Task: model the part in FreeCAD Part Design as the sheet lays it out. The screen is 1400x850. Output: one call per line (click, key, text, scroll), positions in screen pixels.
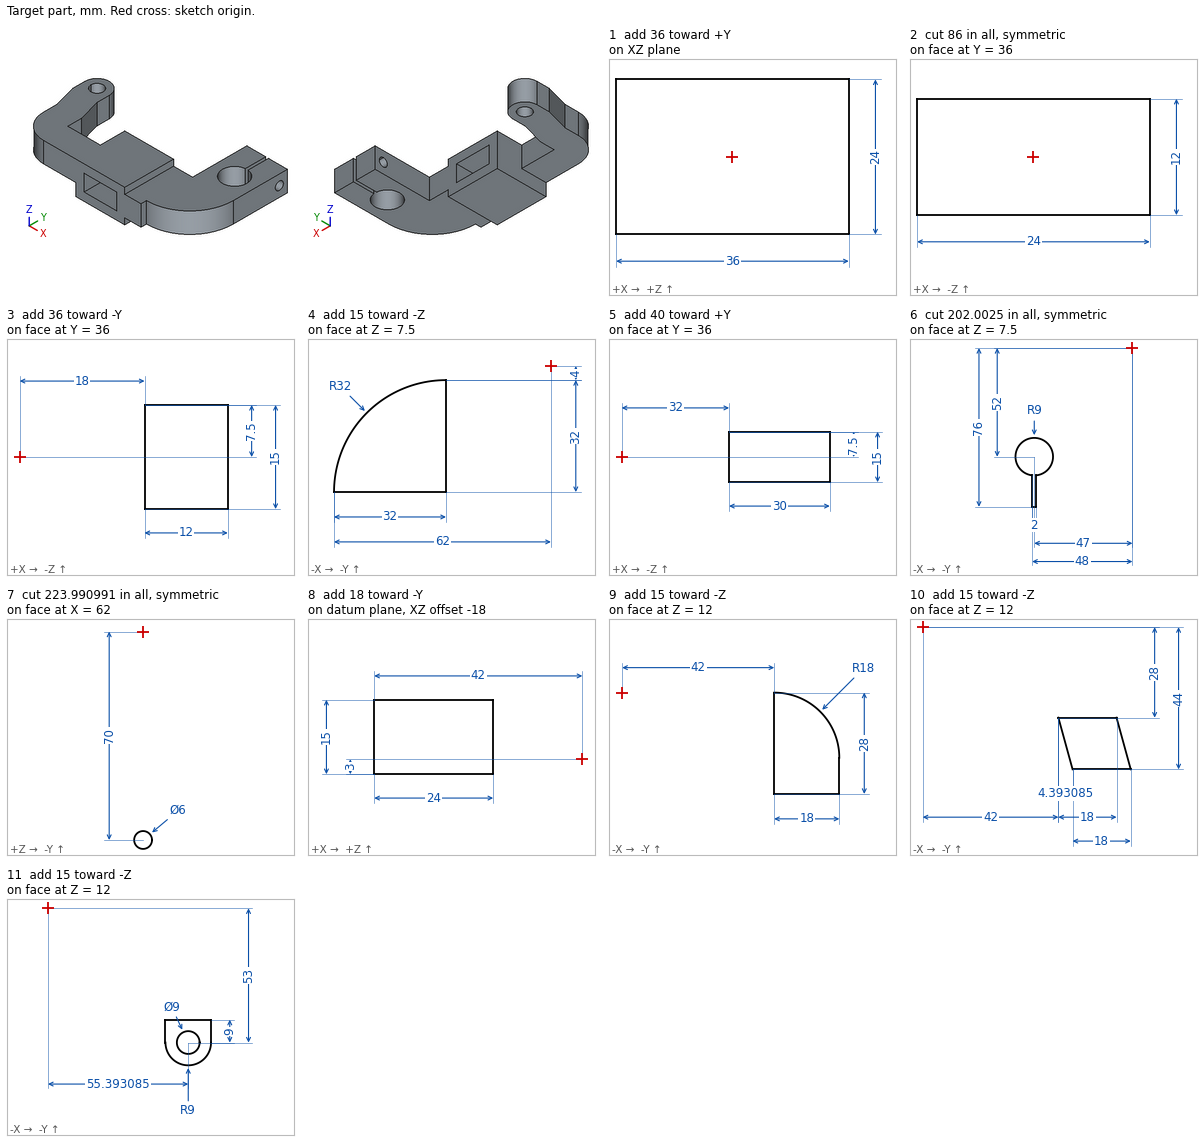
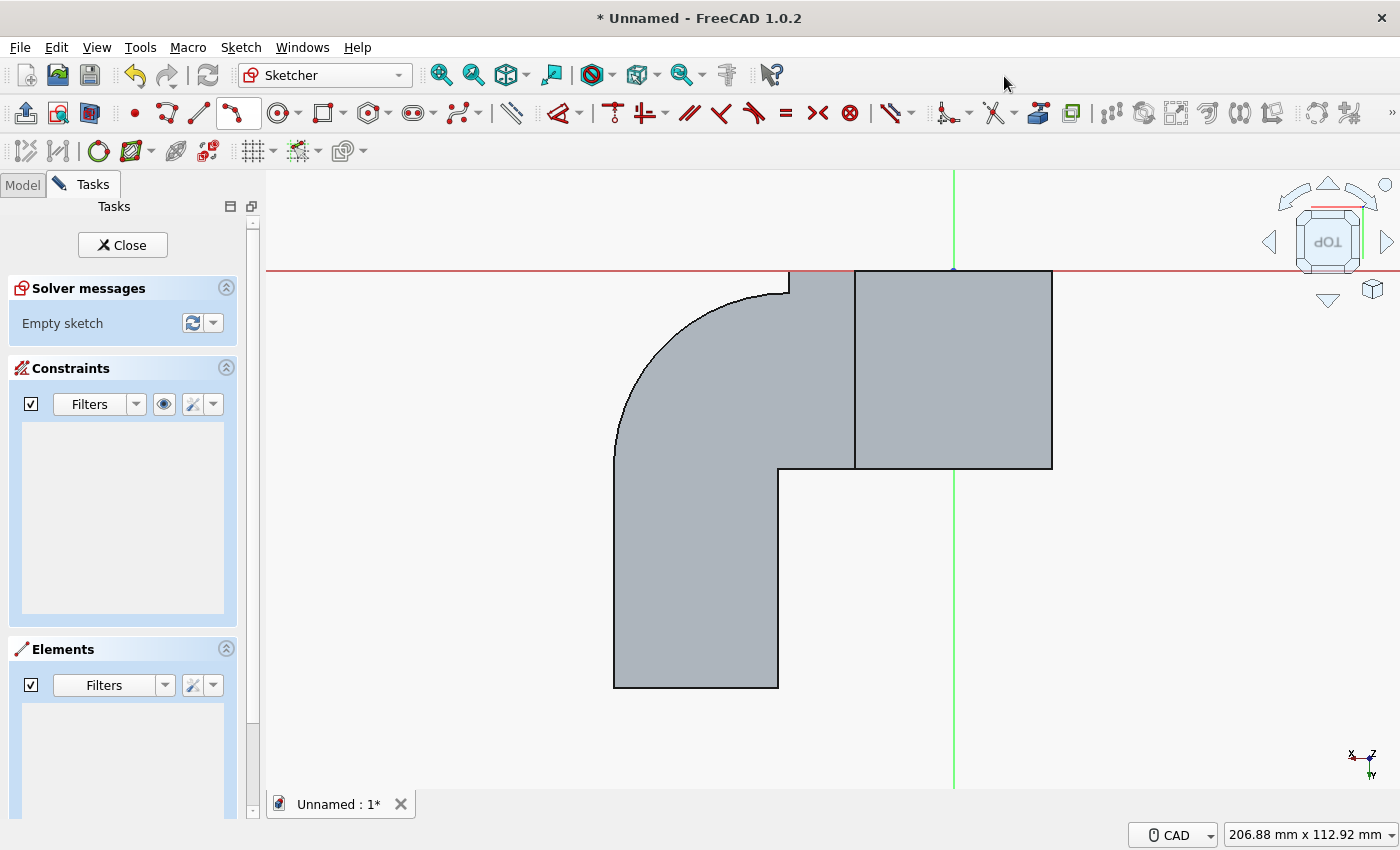
key(q)
key(s)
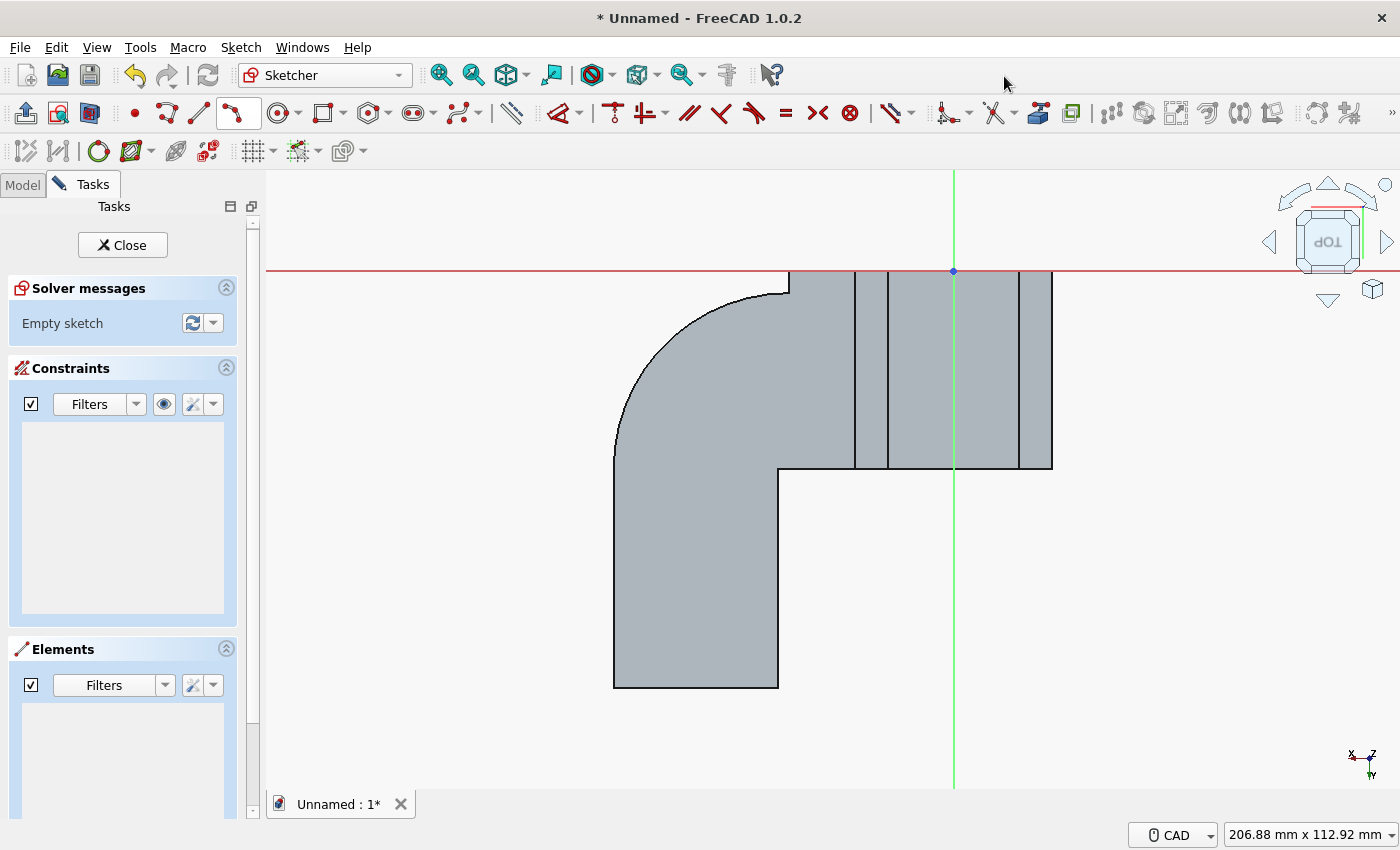
key(g)
key(m)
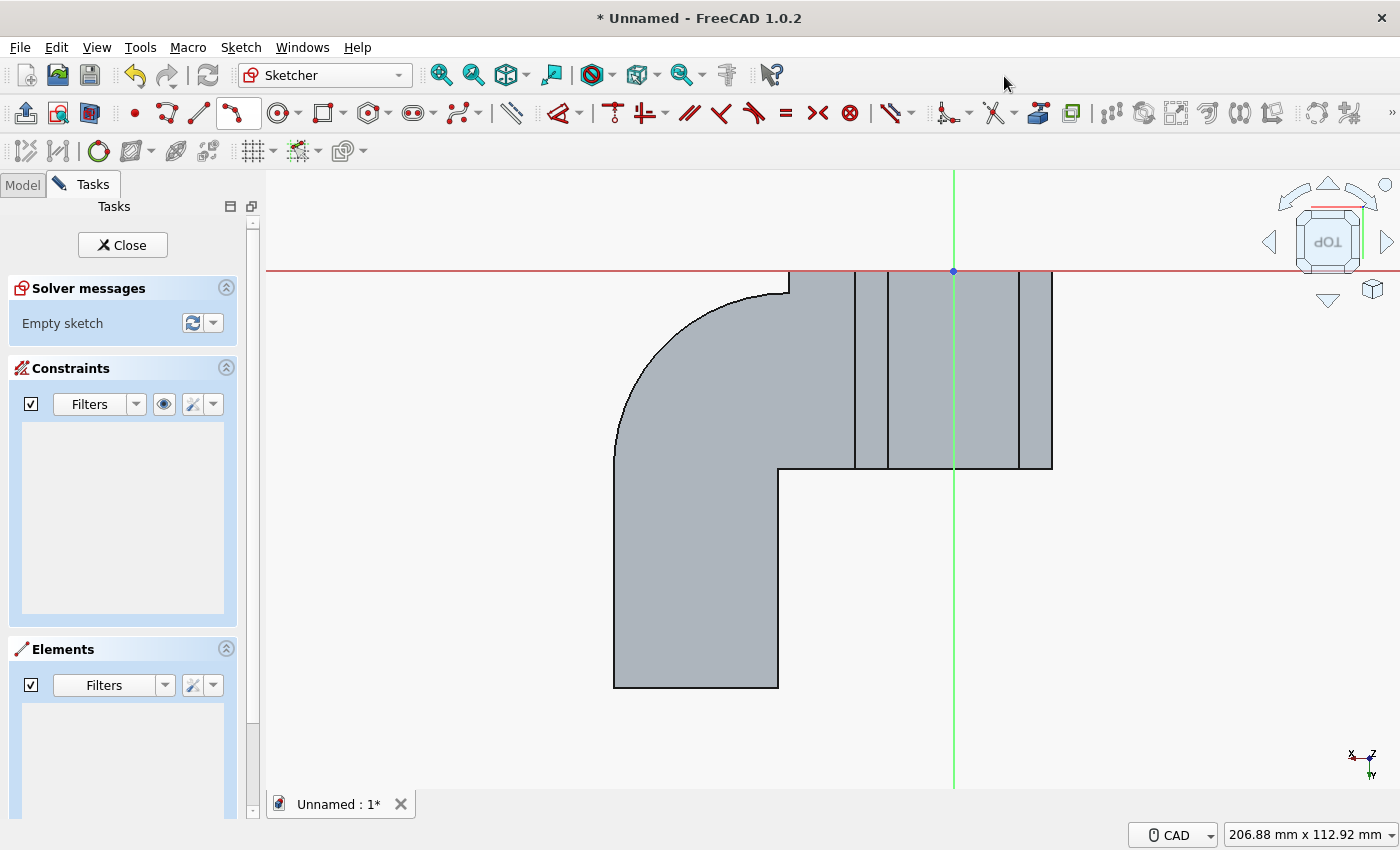
click(690, 605)
click(690, 688)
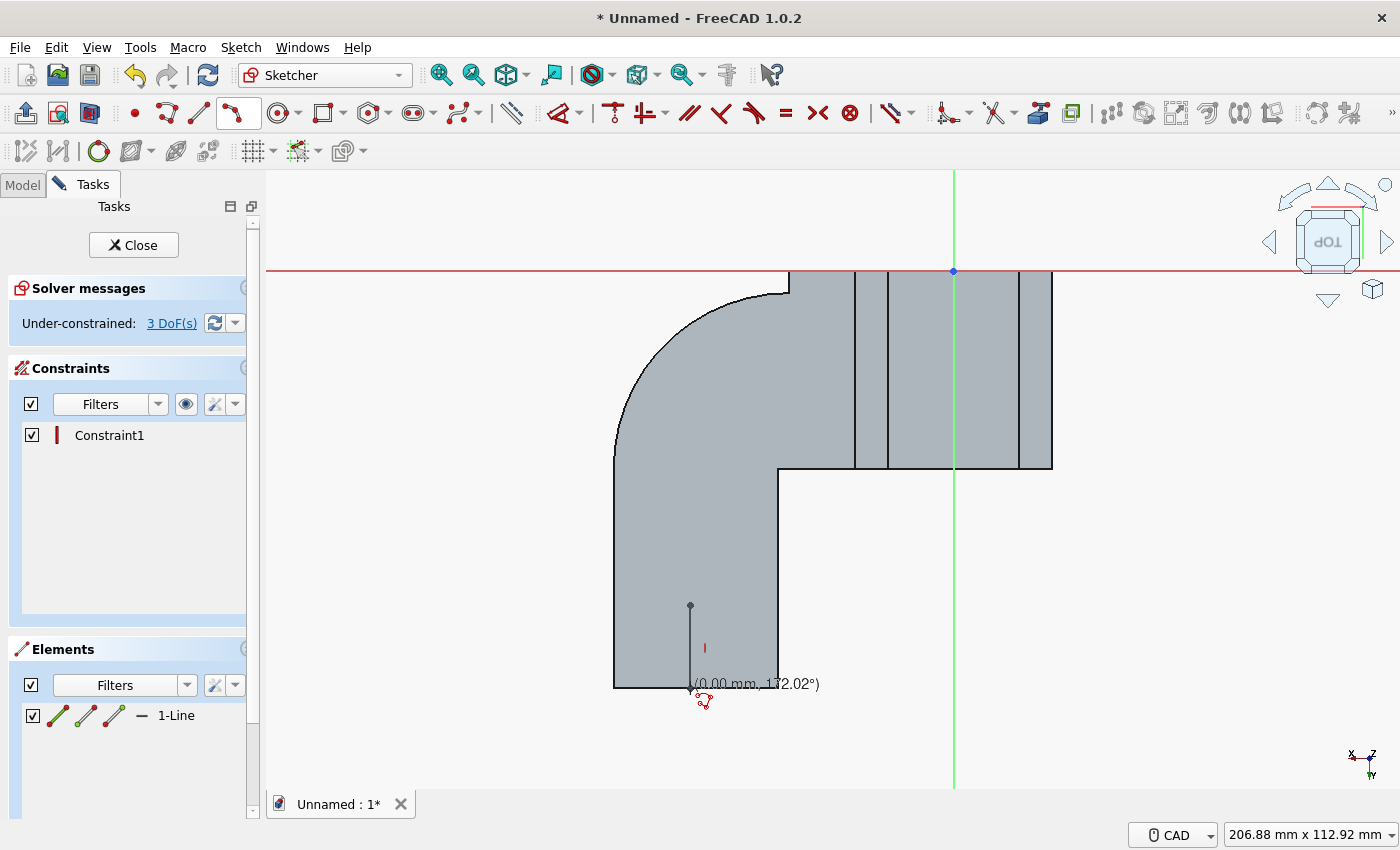
scroll(701, 688, up, 2)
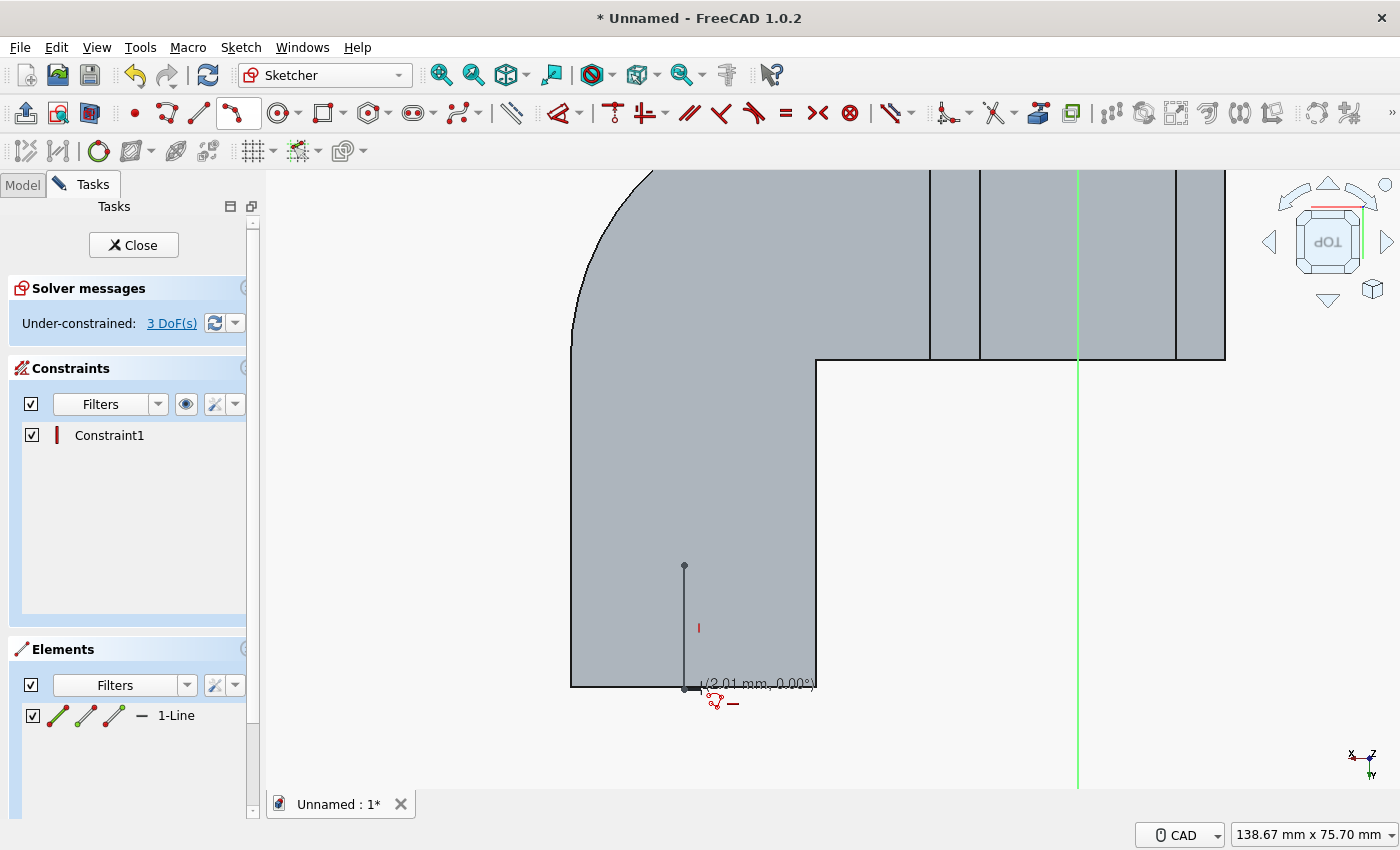
click(701, 688)
click(701, 564)
right_click(701, 564)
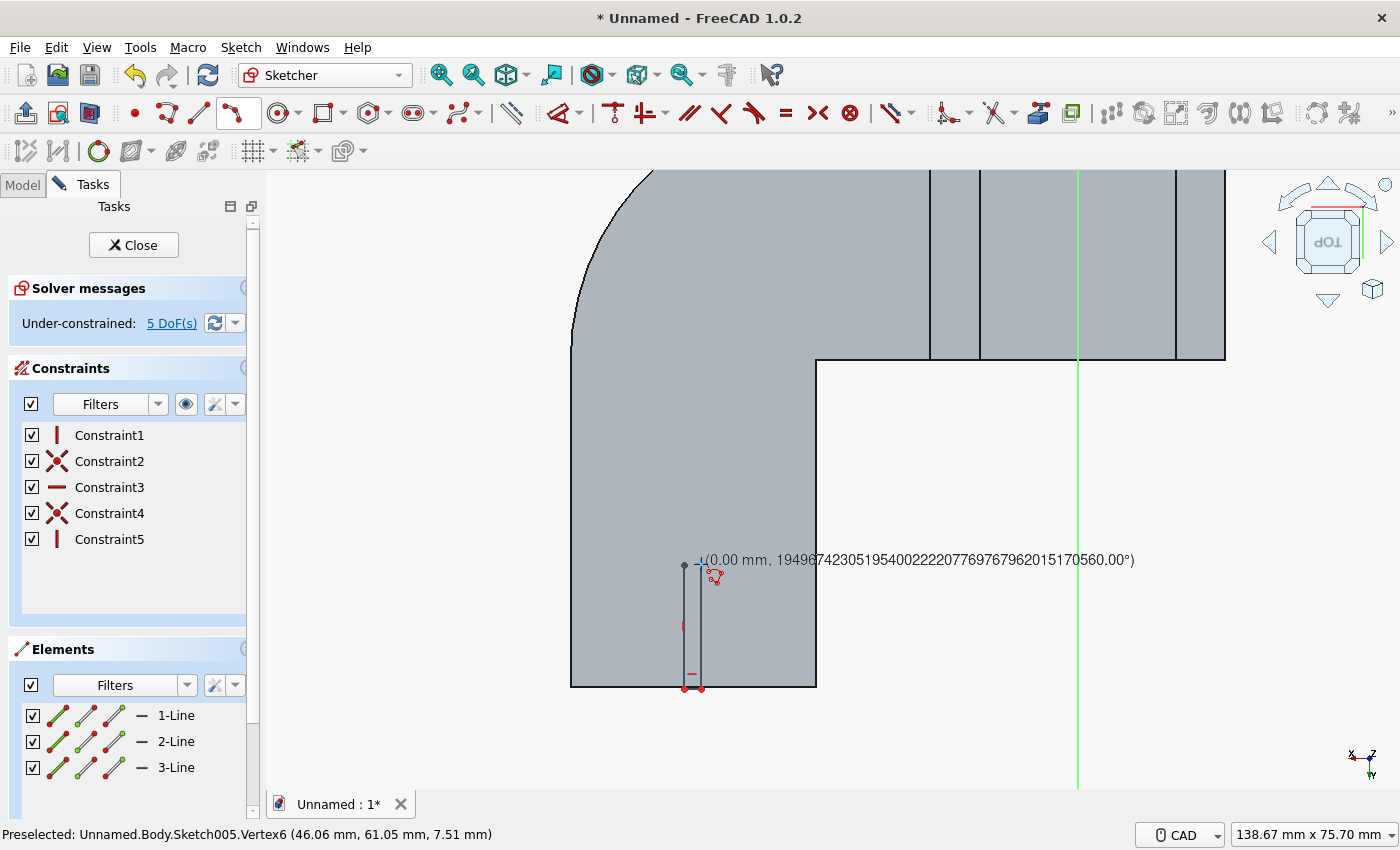
key(g)
key(3)
key(a)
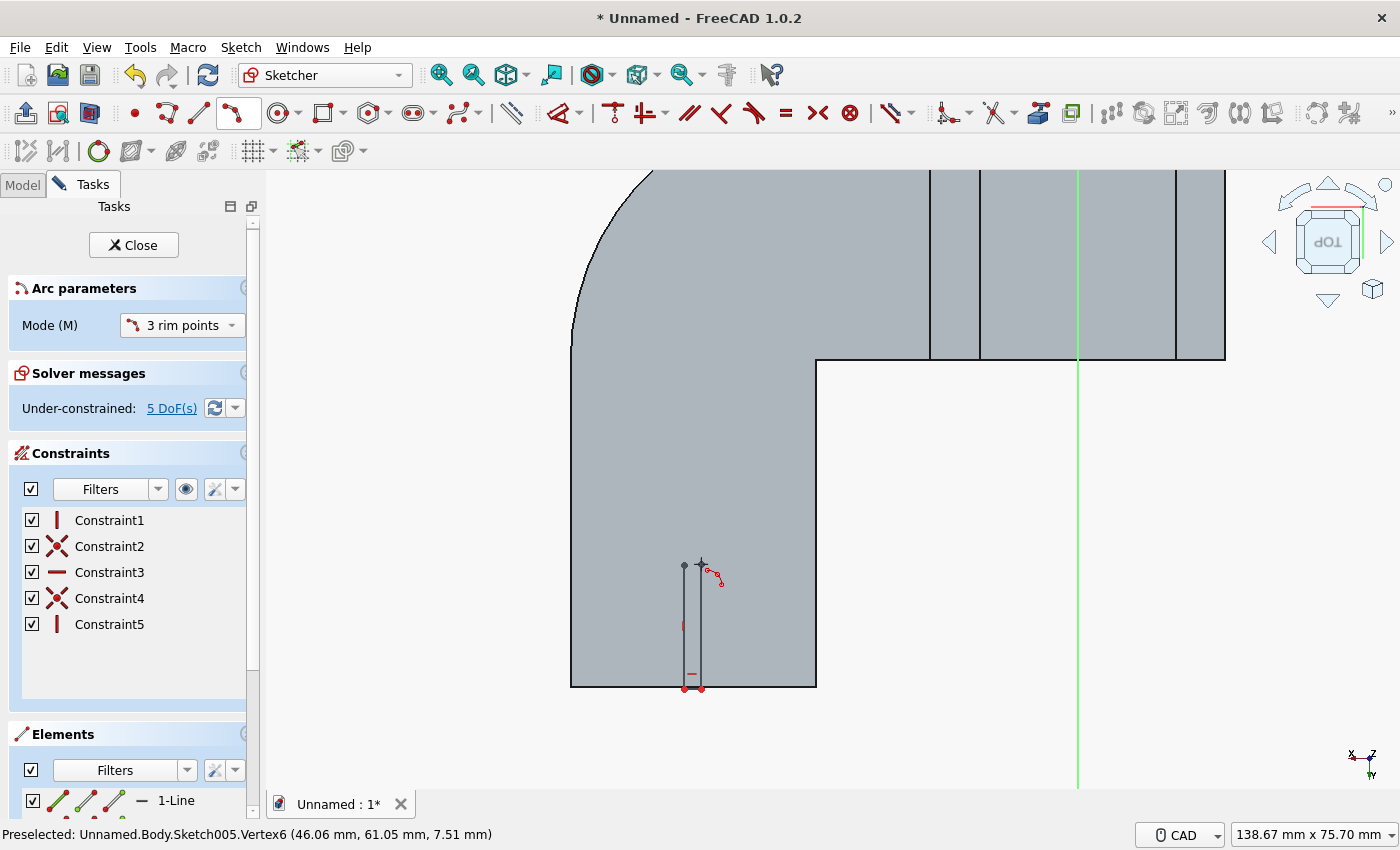
click(701, 565)
click(684, 565)
click(693, 417)
key(Escape)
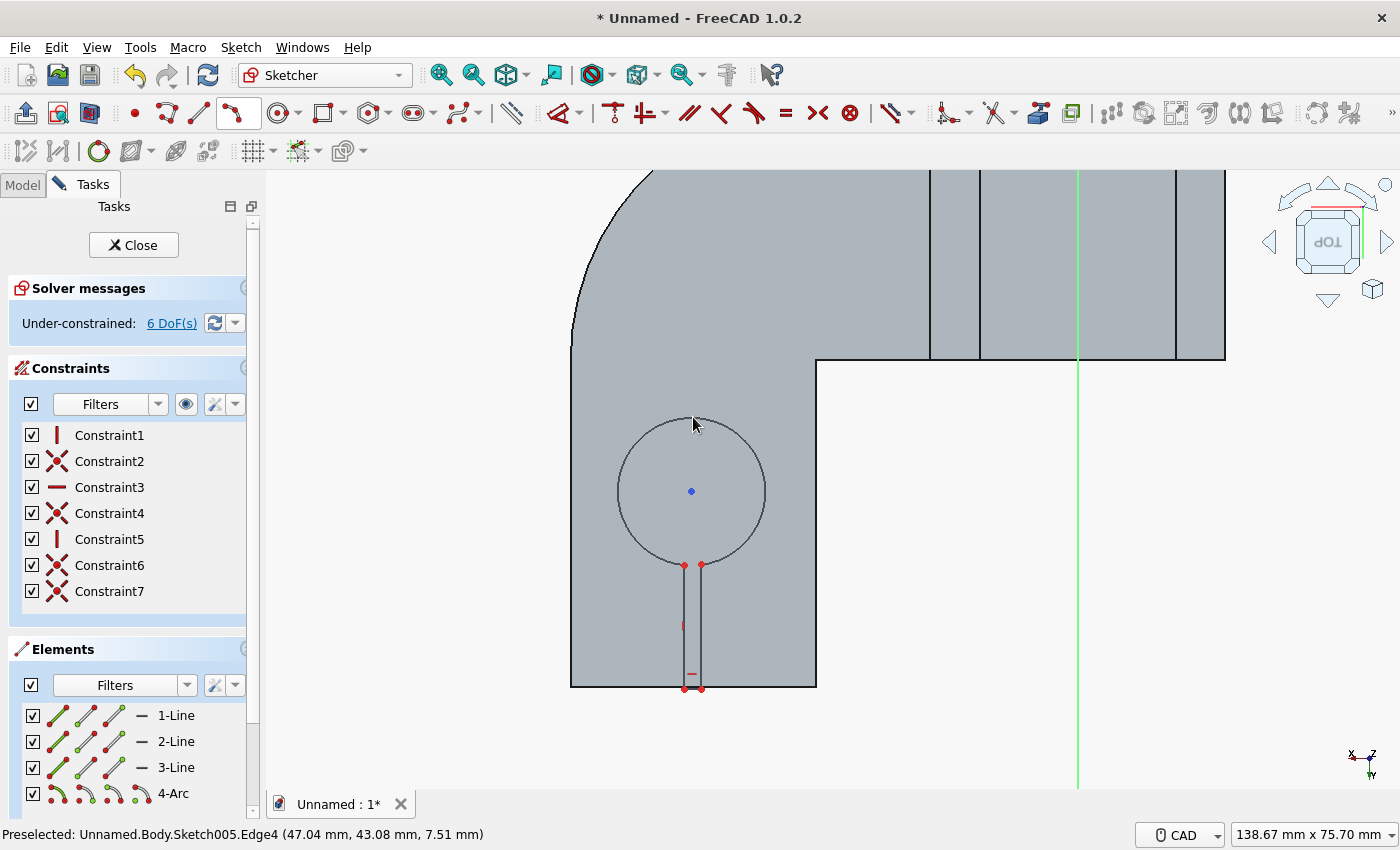
key(d)